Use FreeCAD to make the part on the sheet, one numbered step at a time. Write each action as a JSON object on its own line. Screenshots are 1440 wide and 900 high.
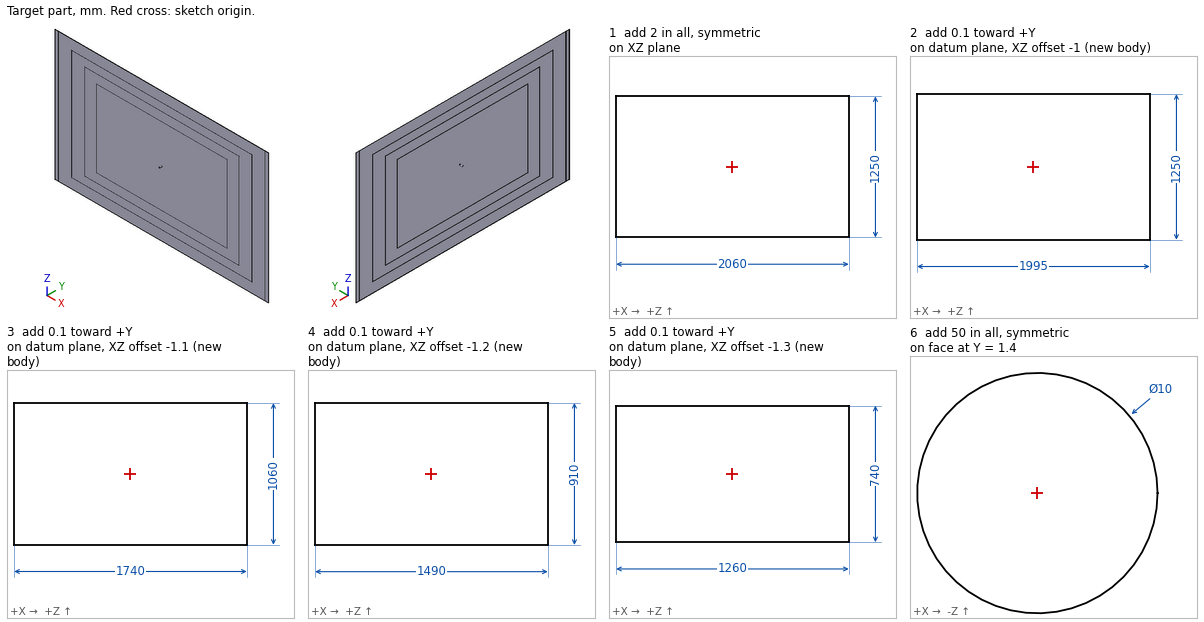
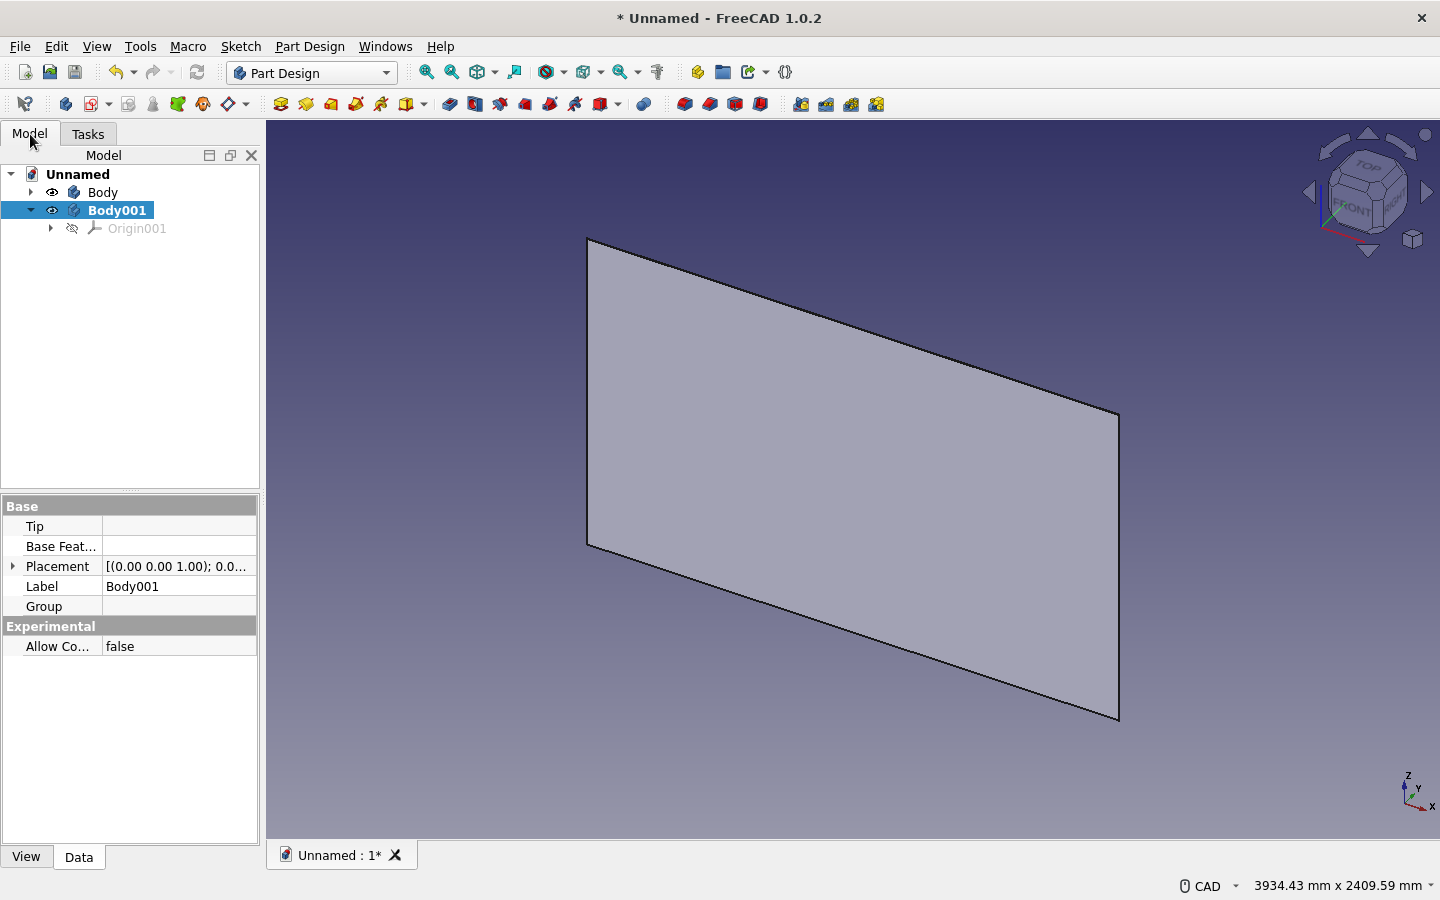
{"action": "left_click", "coordinate": [51, 228]}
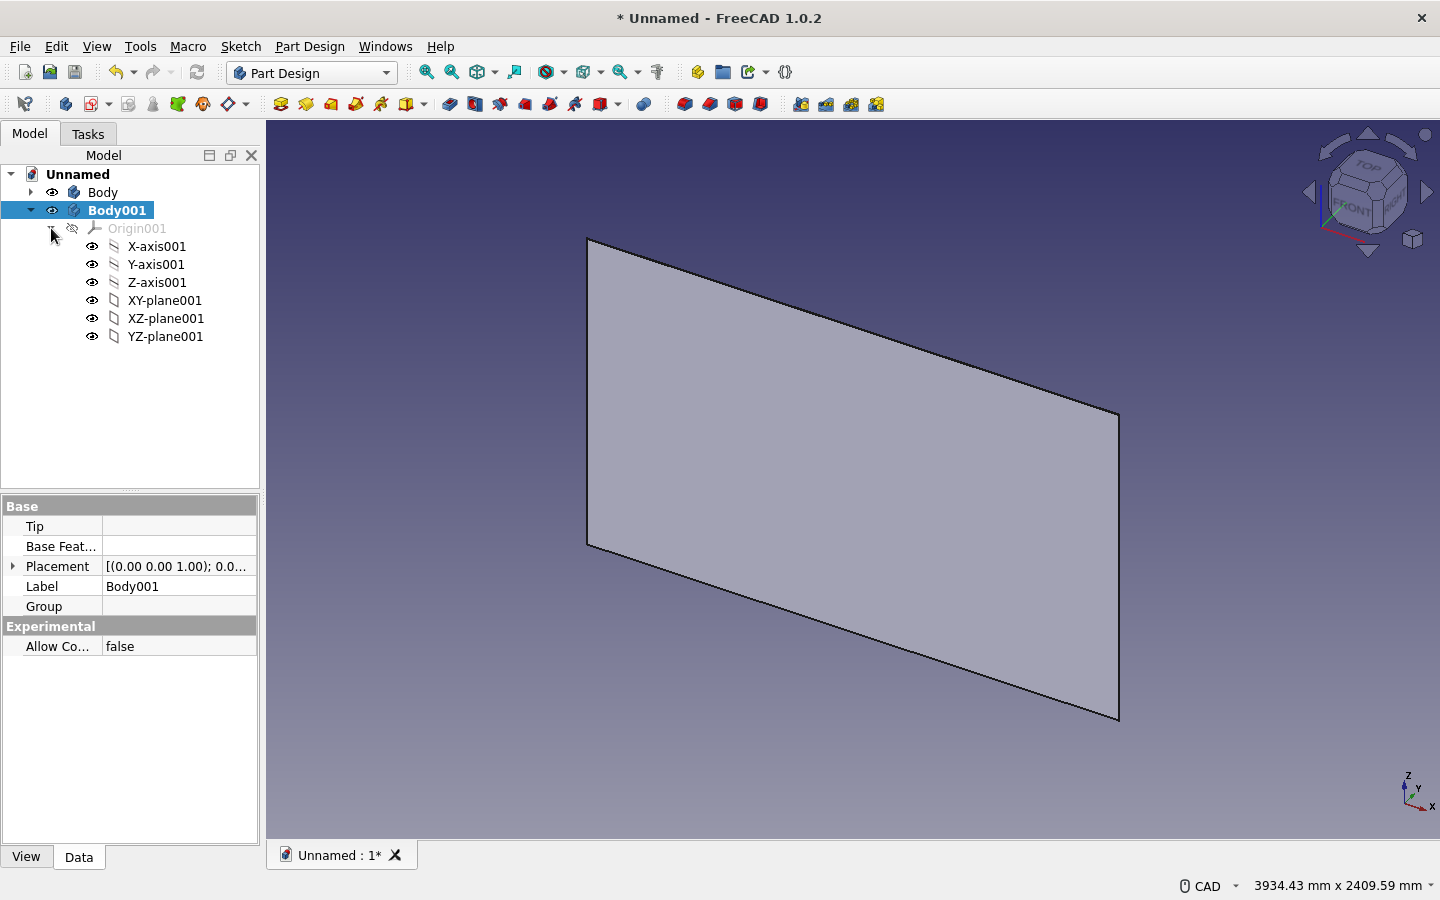
{"action": "left_click", "coordinate": [137, 318]}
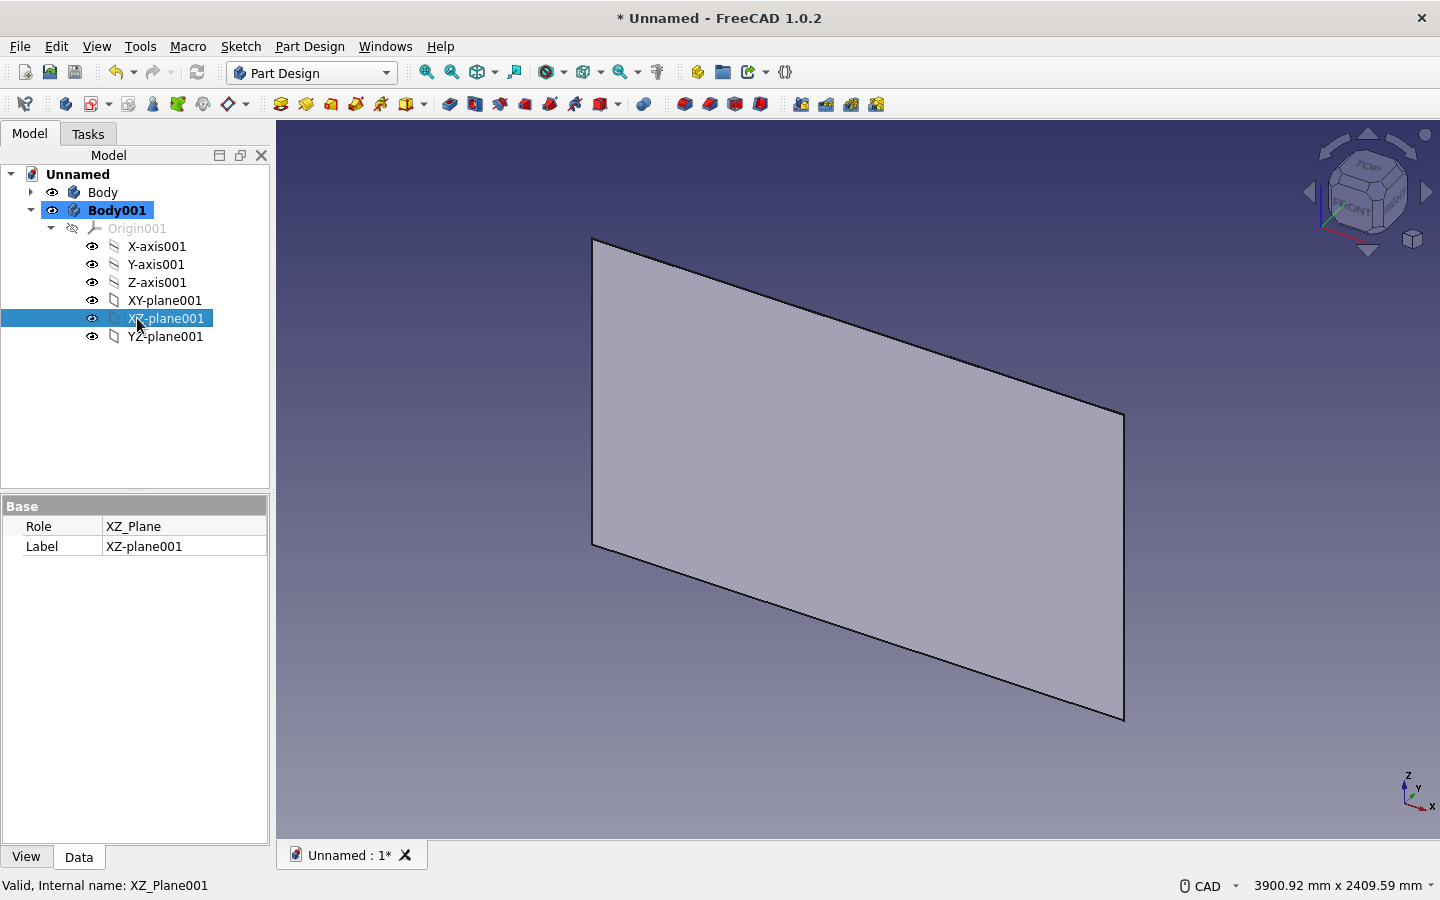
{"action": "left_click", "coordinate": [228, 104]}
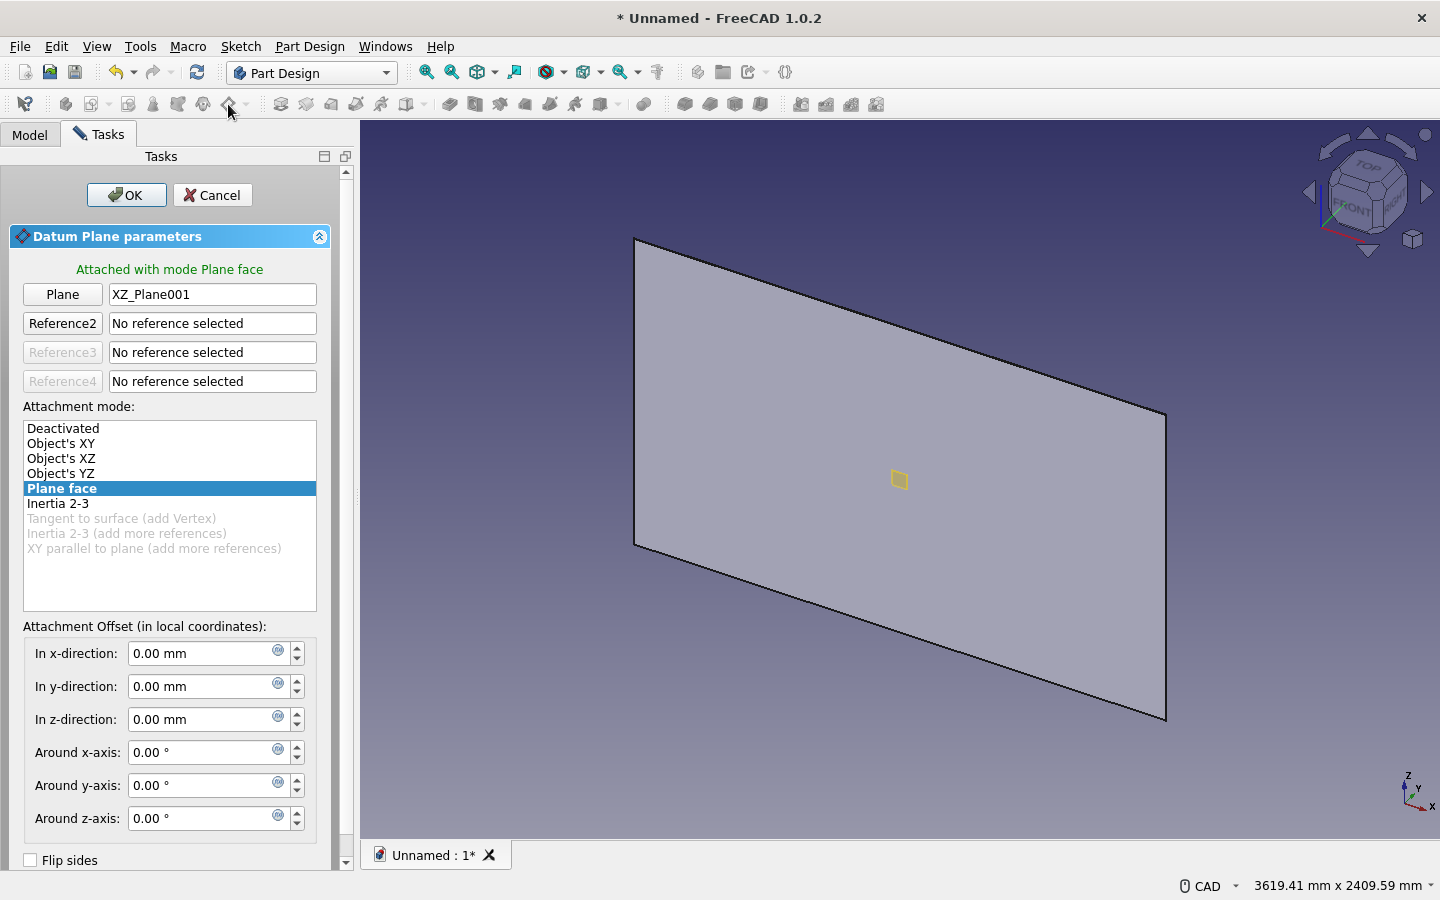
{"action": "triple_click", "coordinate": [210, 720]}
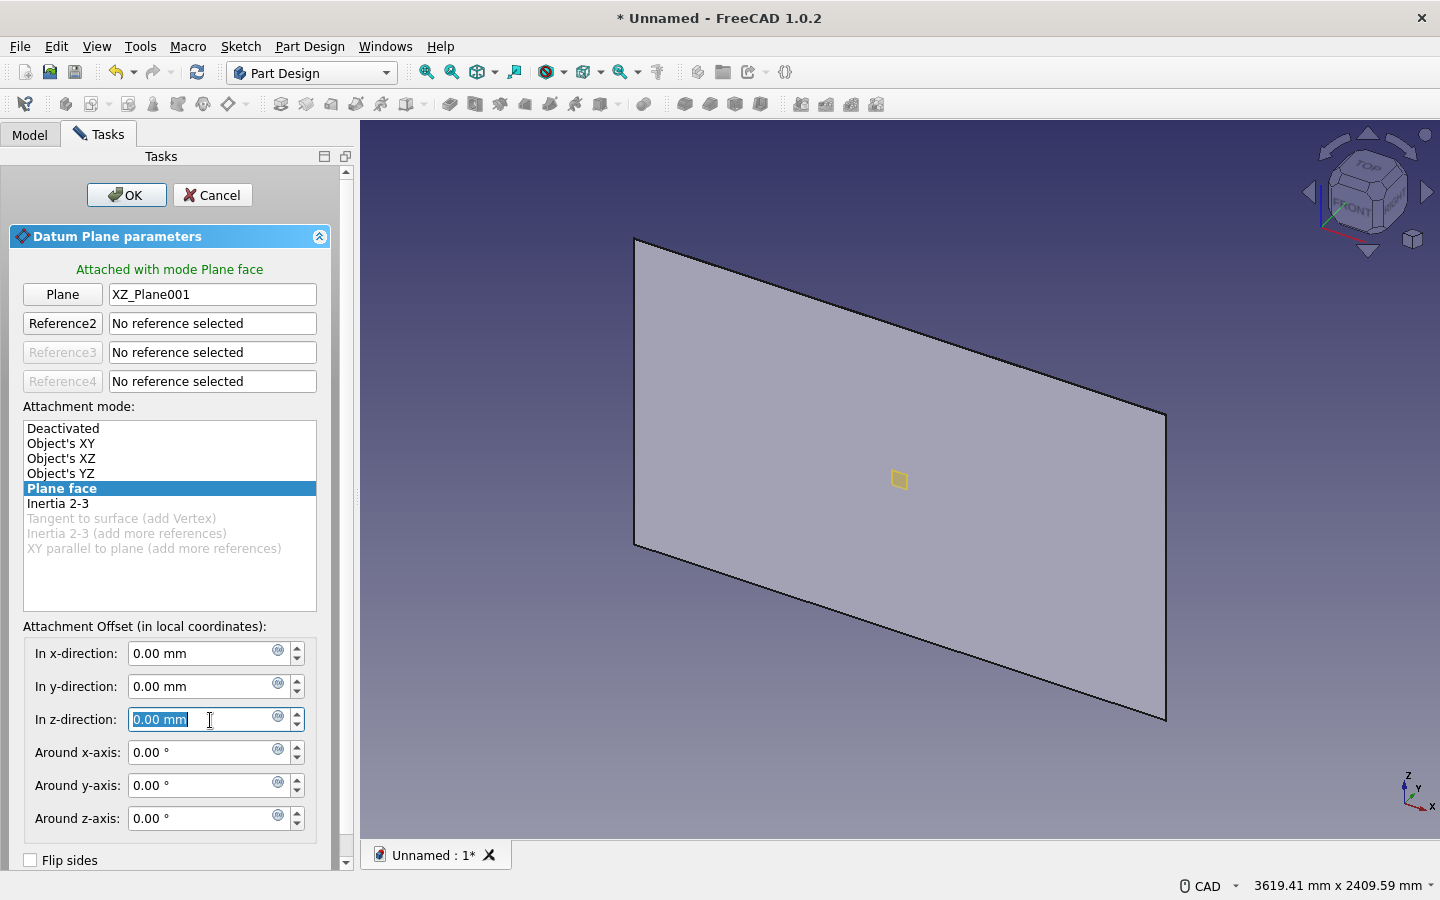
{"action": "type", "text": "-1"}
{"action": "key", "text": "Tab"}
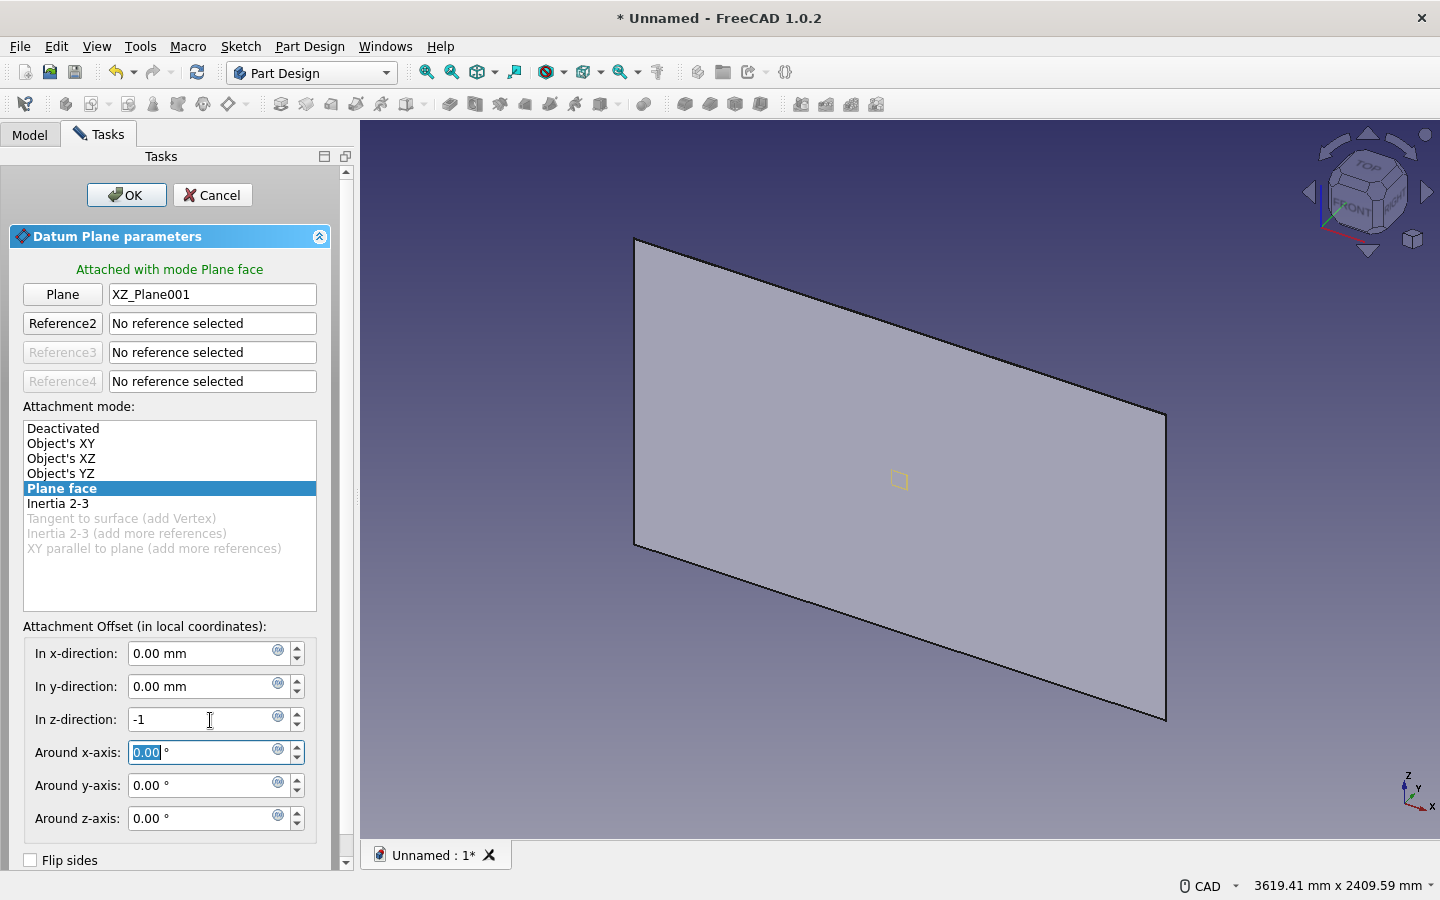
{"action": "left_click", "coordinate": [127, 195]}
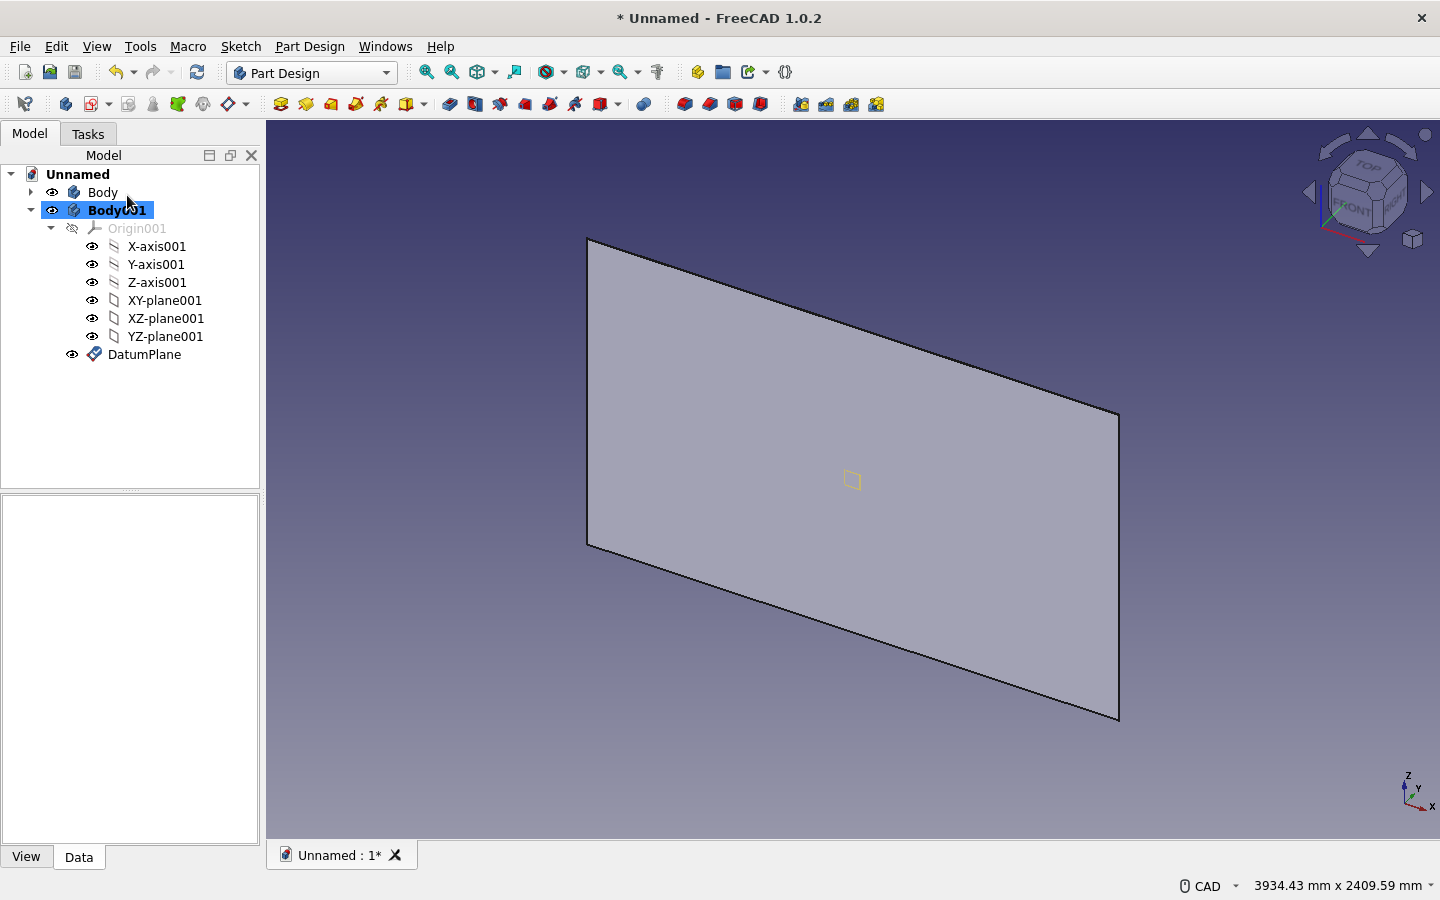
{"action": "left_click", "coordinate": [117, 354]}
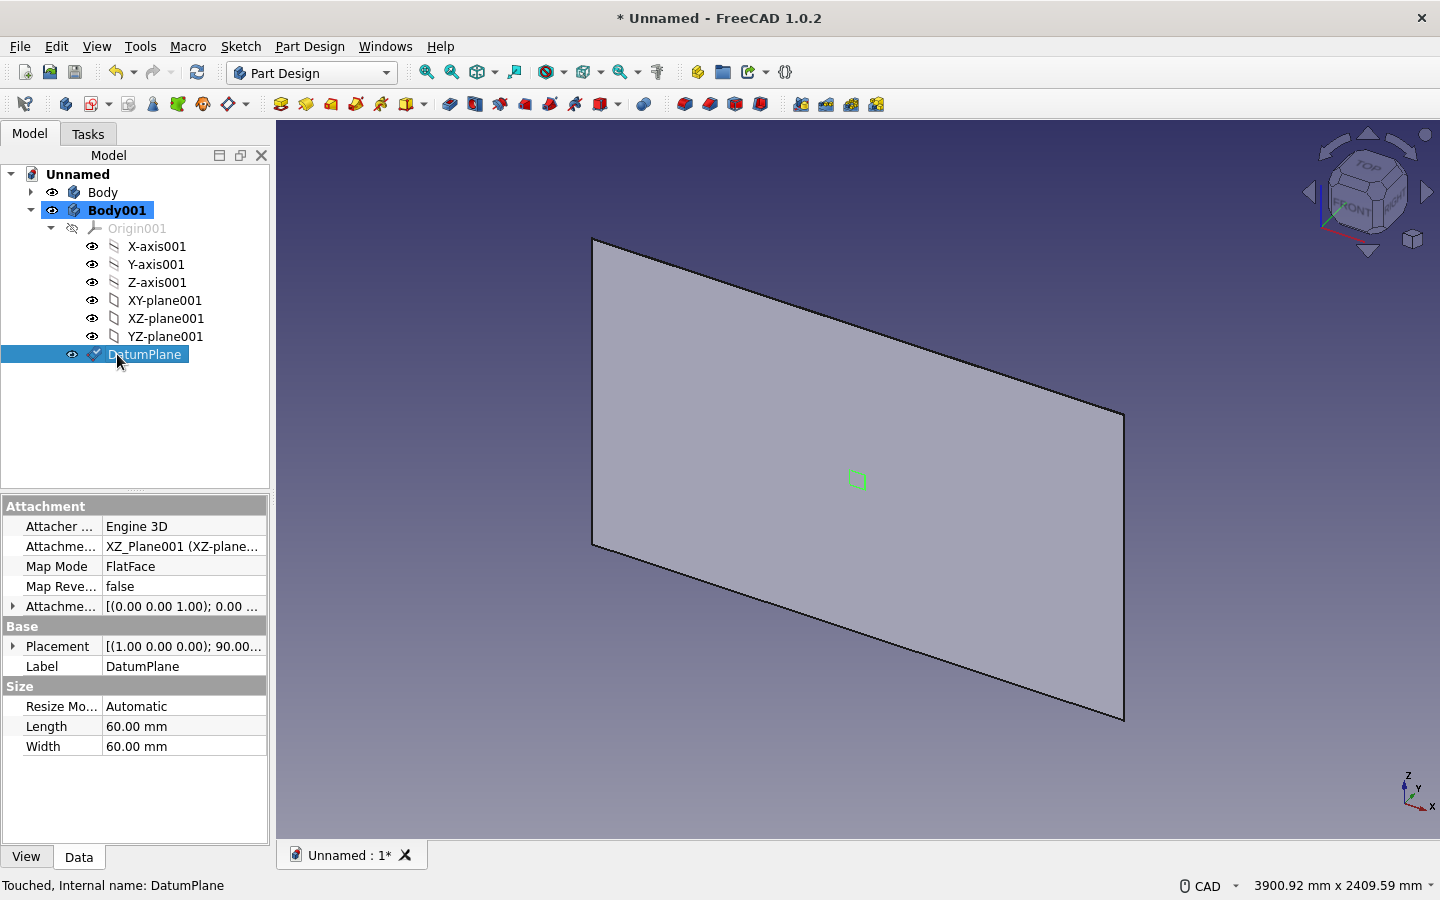
{"action": "left_click", "coordinate": [90, 104]}